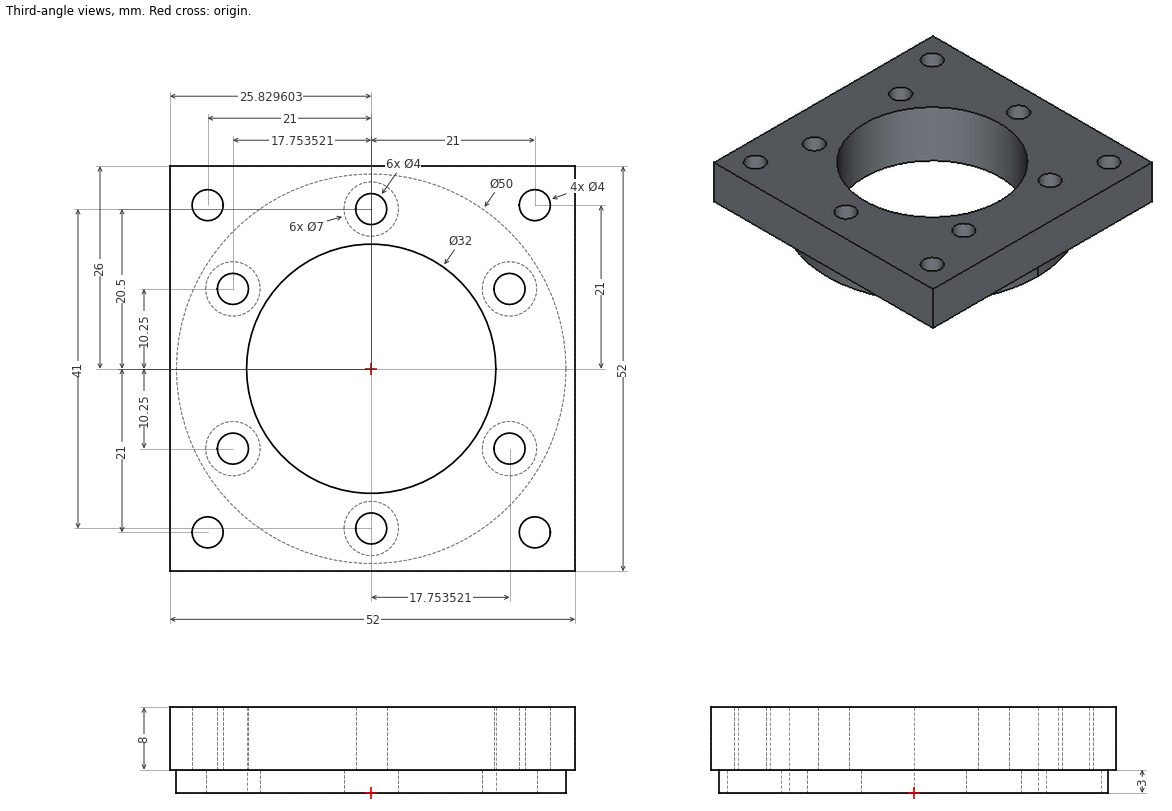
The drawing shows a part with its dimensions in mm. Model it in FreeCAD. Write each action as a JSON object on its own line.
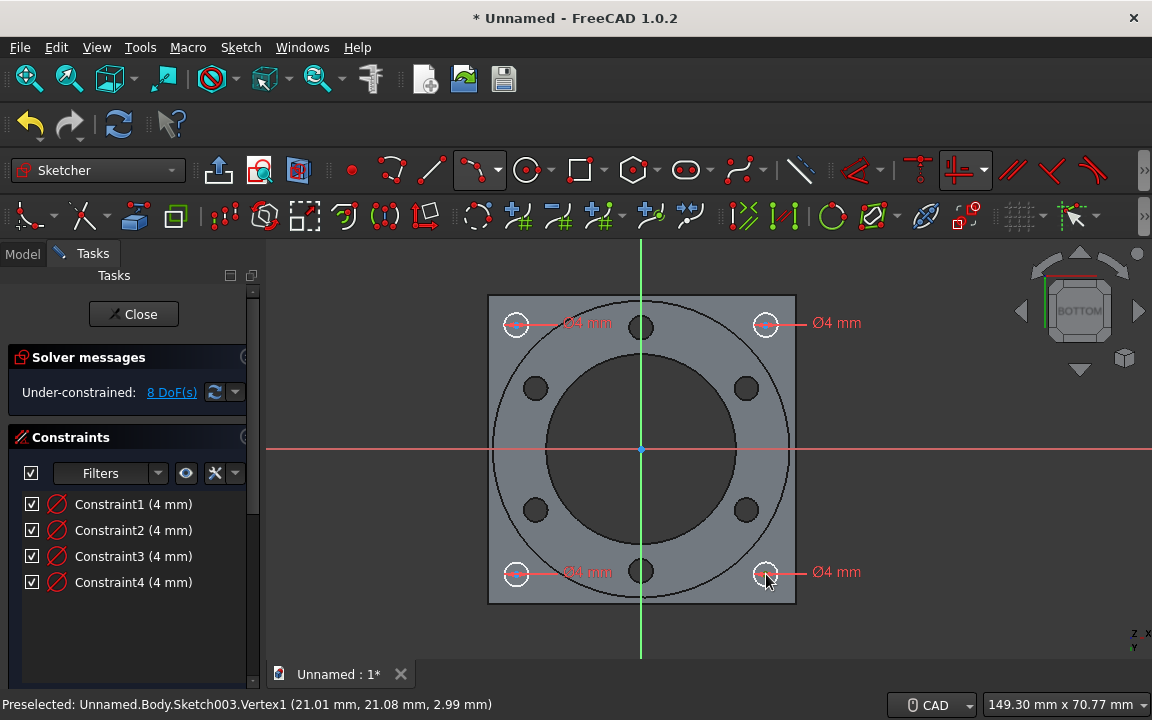
{"action": "left_click", "coordinate": [517, 574]}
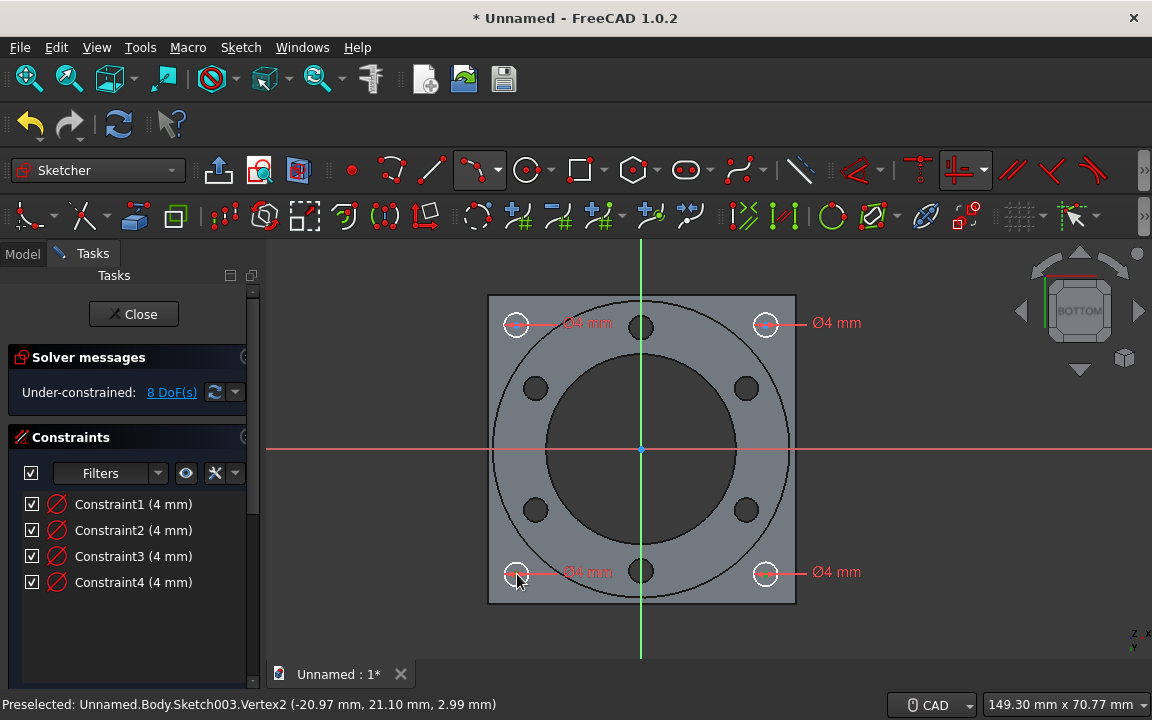
{"action": "key", "text": "h"}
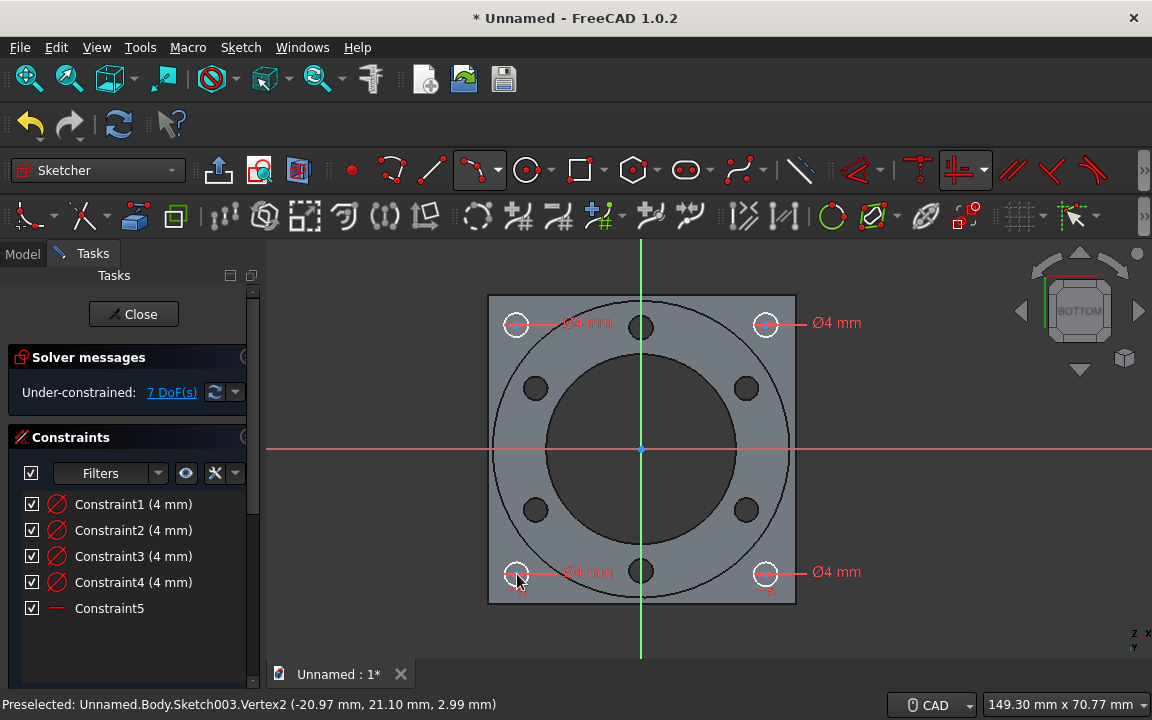
{"action": "left_click", "coordinate": [517, 574]}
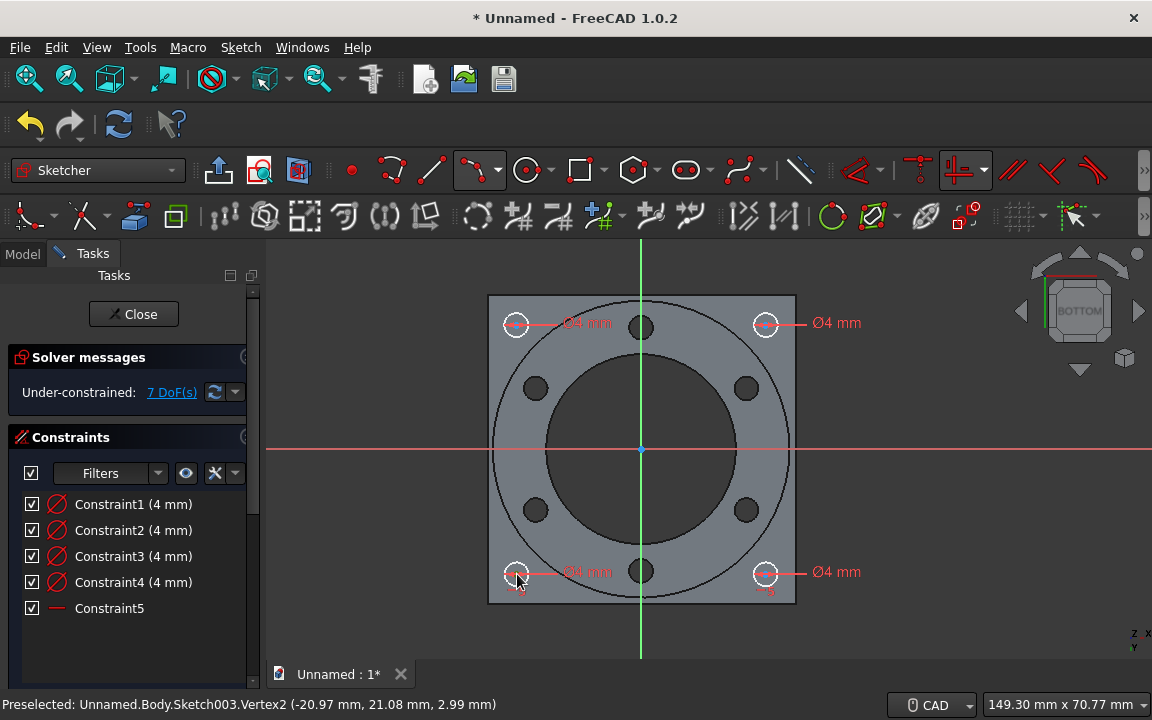
{"action": "left_click", "coordinate": [516, 325]}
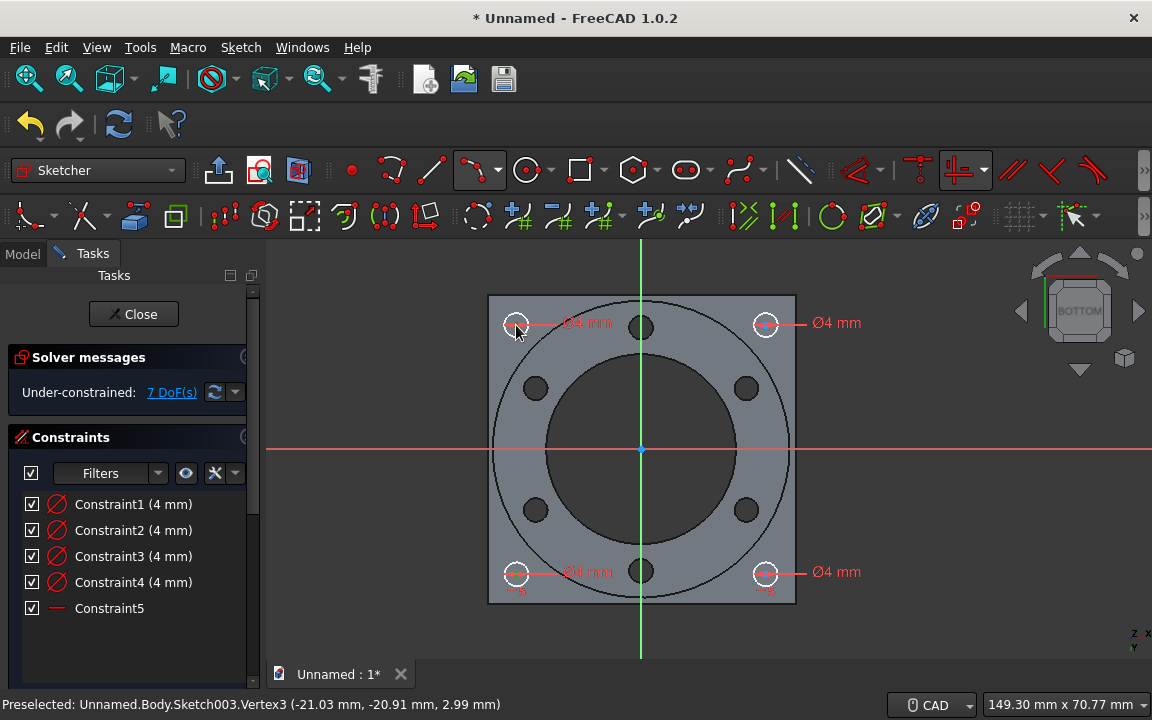
{"action": "key", "text": "v"}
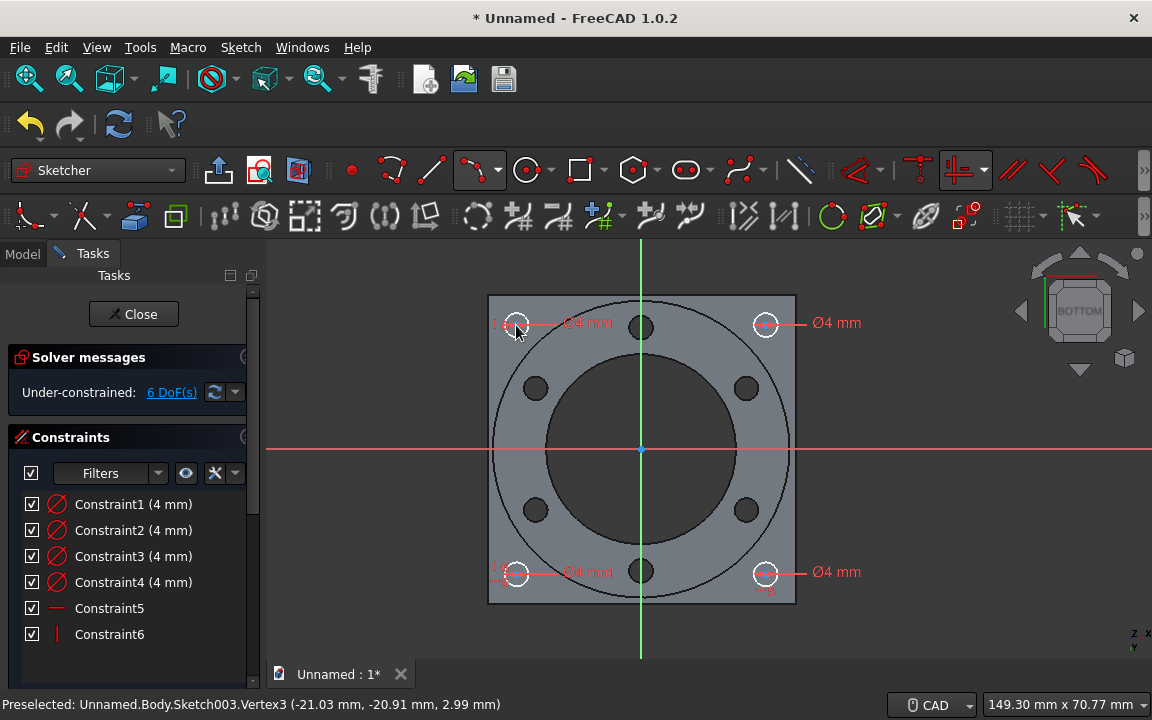
{"action": "left_click", "coordinate": [766, 574]}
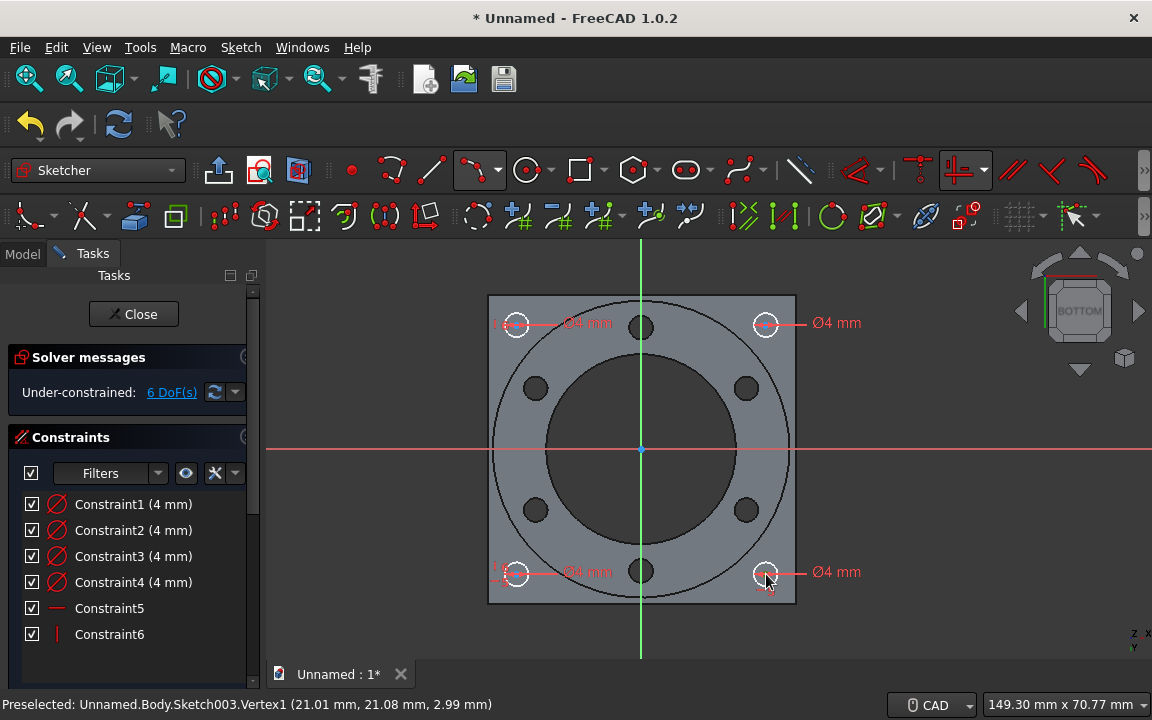
{"action": "left_click", "coordinate": [766, 325]}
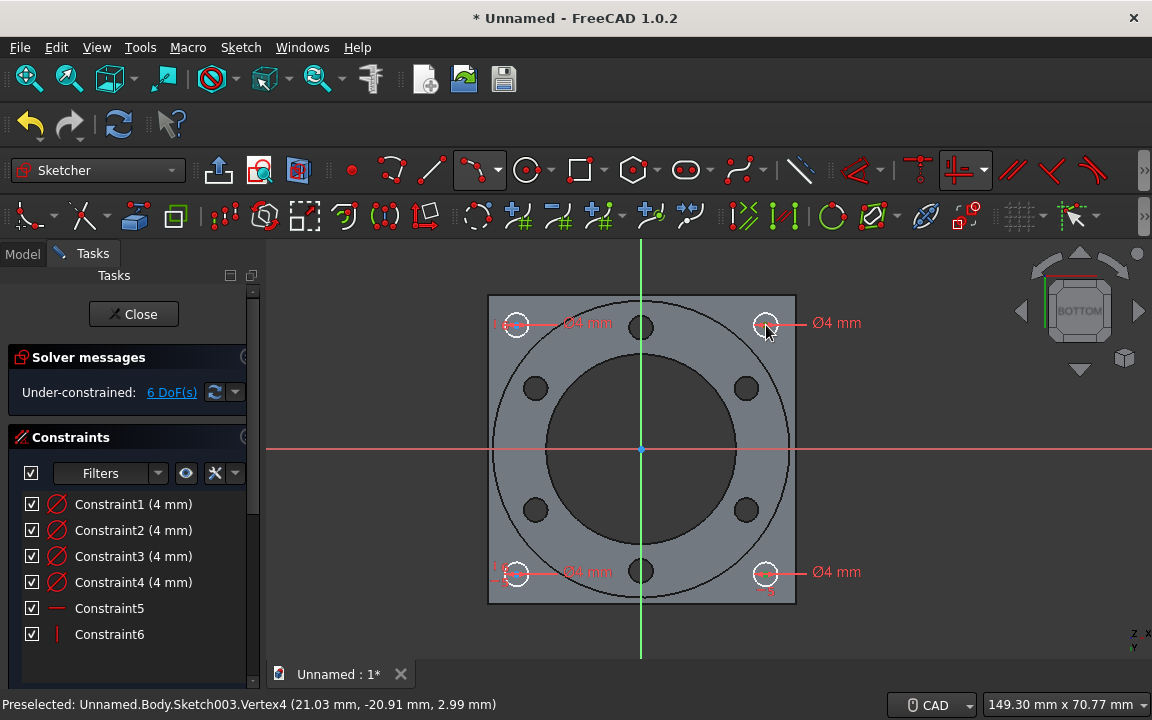
{"action": "key", "text": "v"}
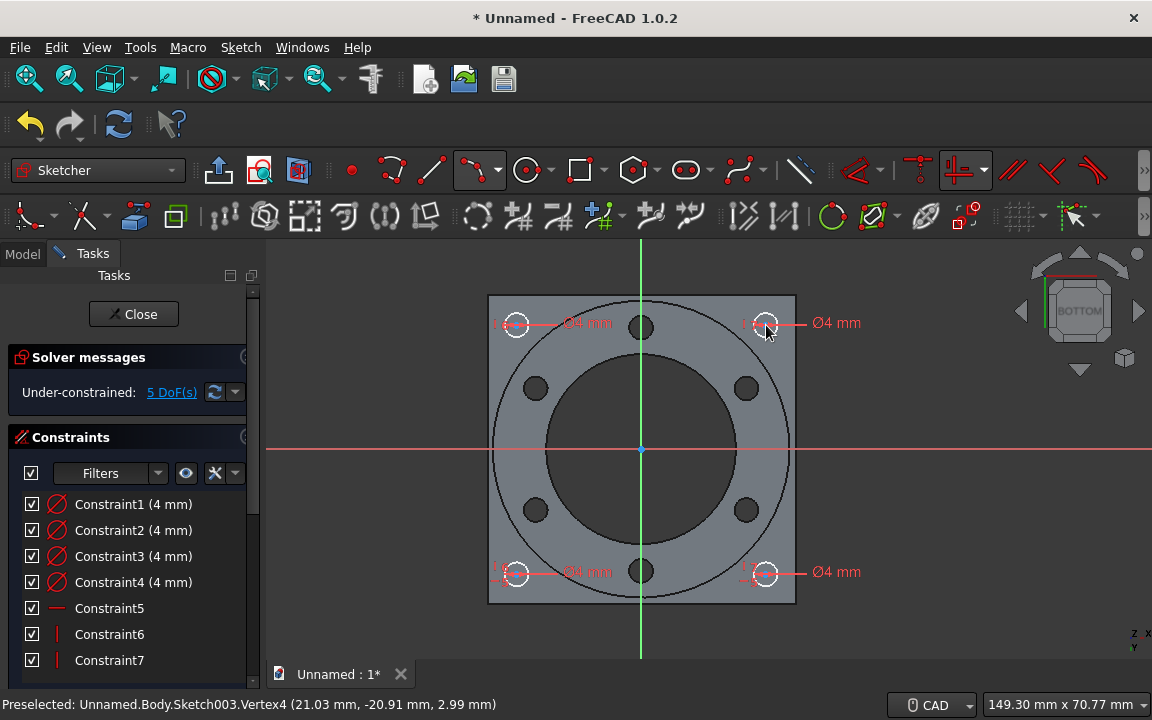
{"action": "left_click", "coordinate": [517, 325]}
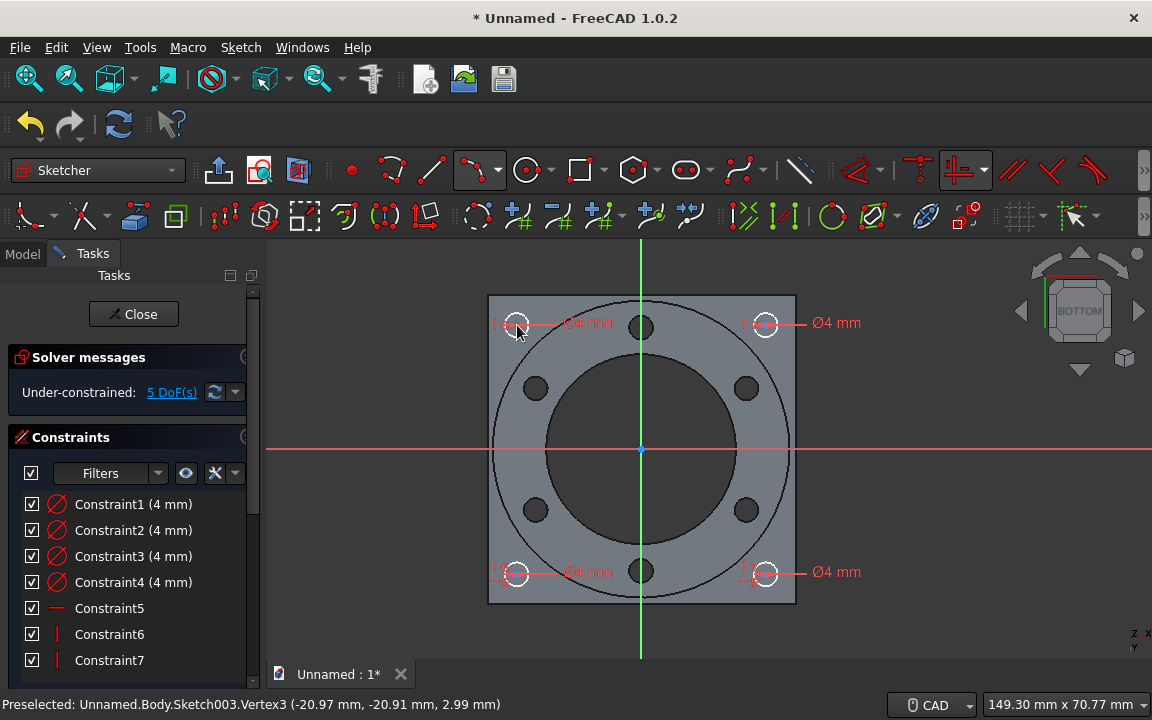
{"action": "left_click", "coordinate": [766, 325]}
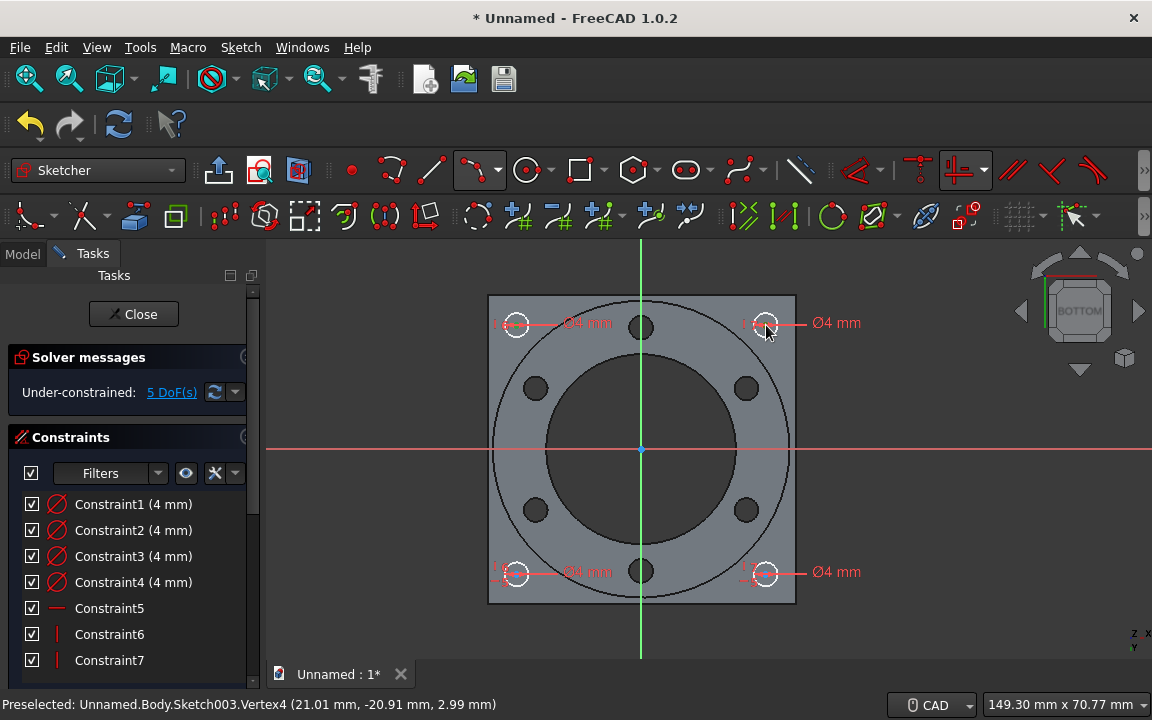
{"action": "key", "text": "h"}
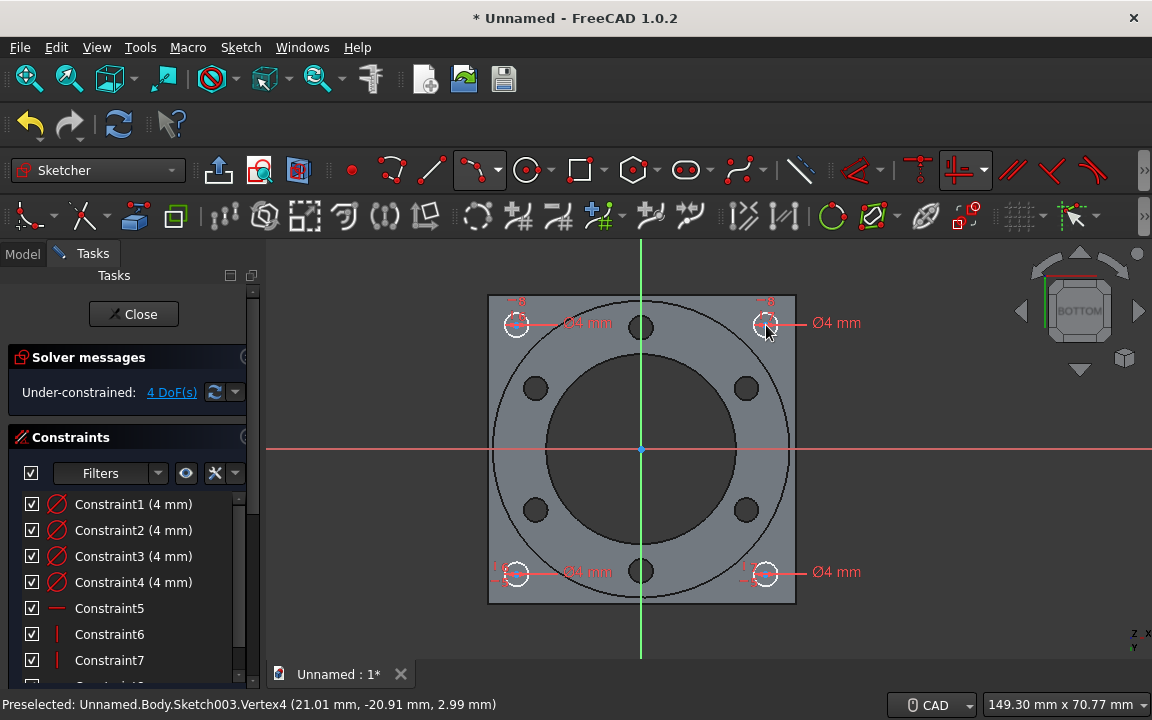
{"action": "left_click", "coordinate": [856, 170]}